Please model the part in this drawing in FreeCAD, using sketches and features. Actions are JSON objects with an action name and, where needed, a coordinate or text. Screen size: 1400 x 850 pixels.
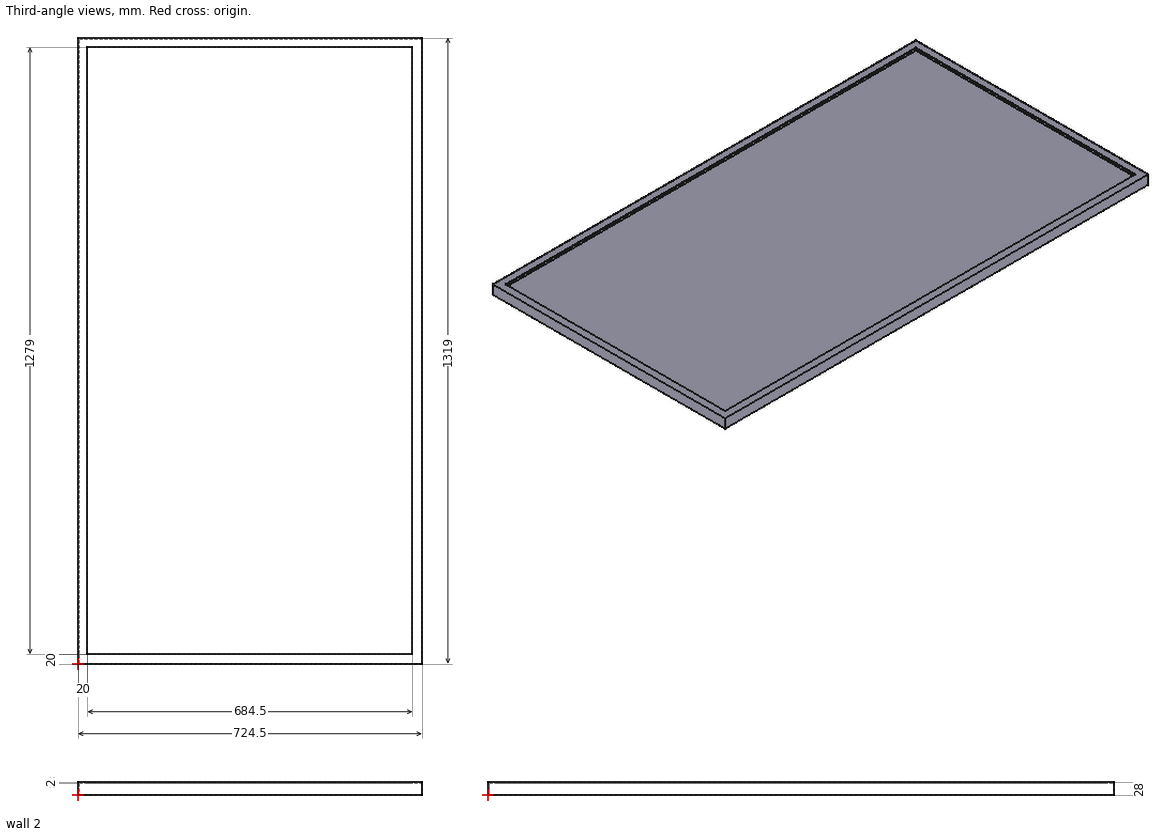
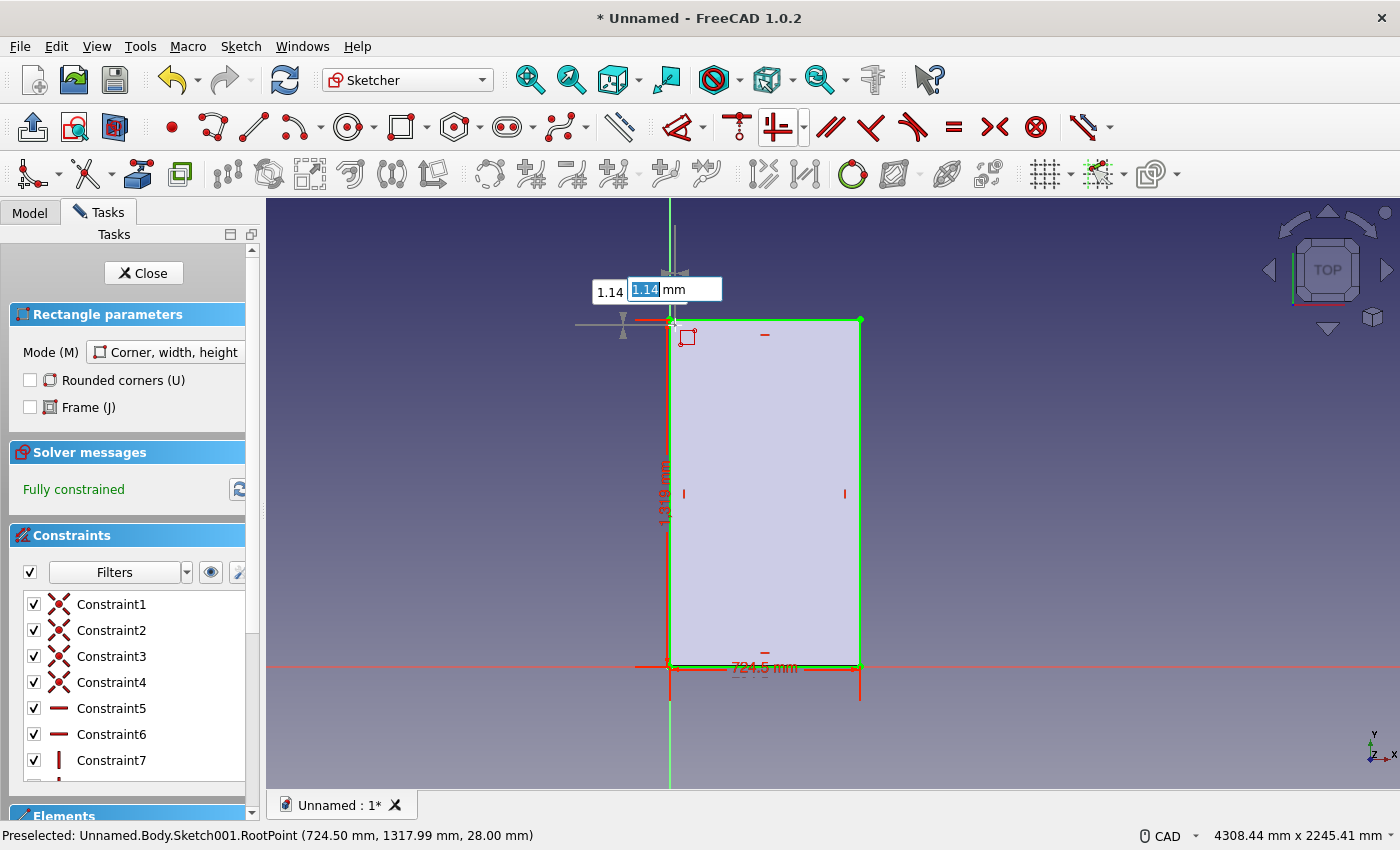
{"action": "scroll", "coordinate": [855, 662], "scroll_direction": "up", "scroll_amount": 6}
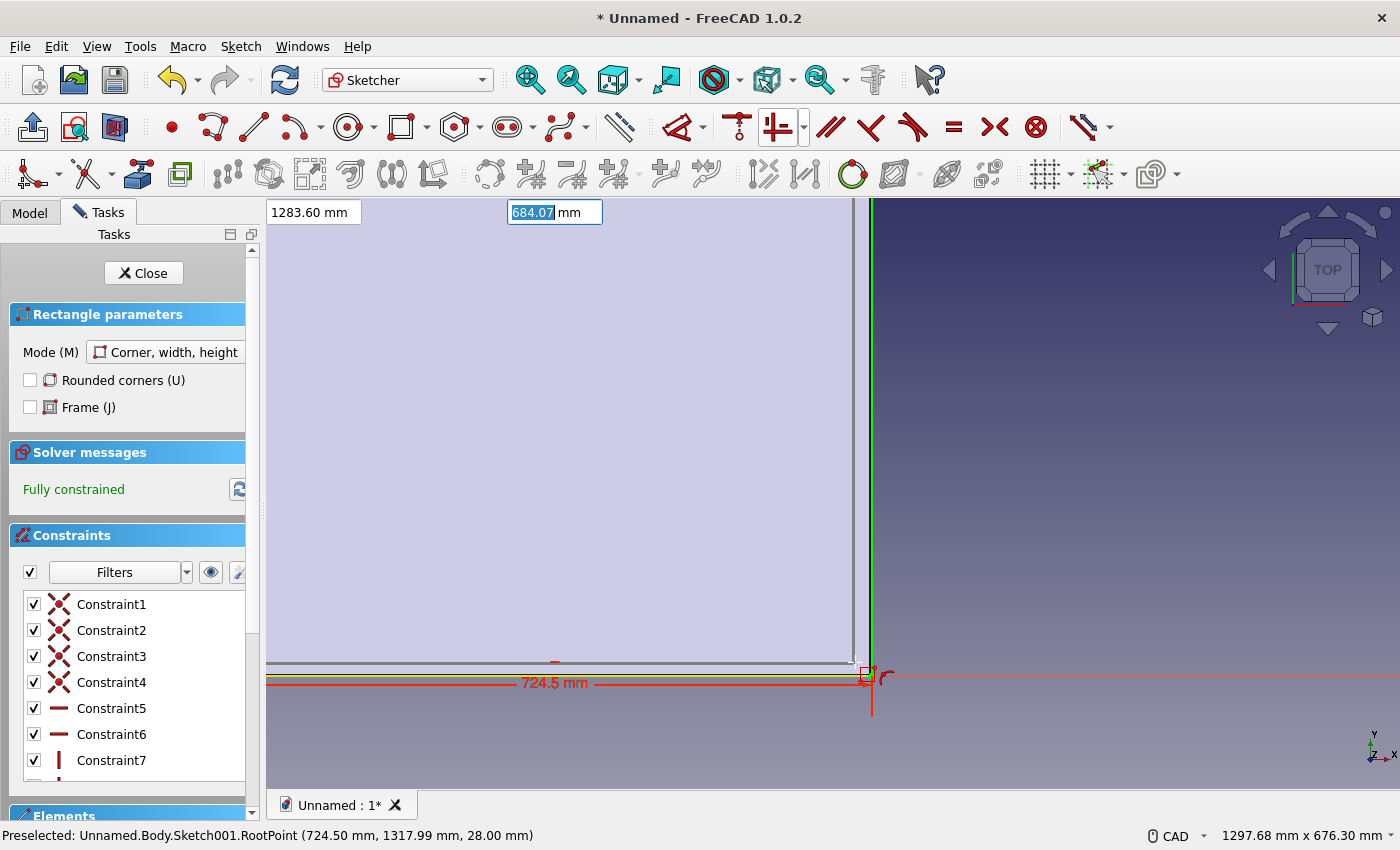
{"action": "left_click", "coordinate": [854, 659]}
{"action": "key", "text": "Escape"}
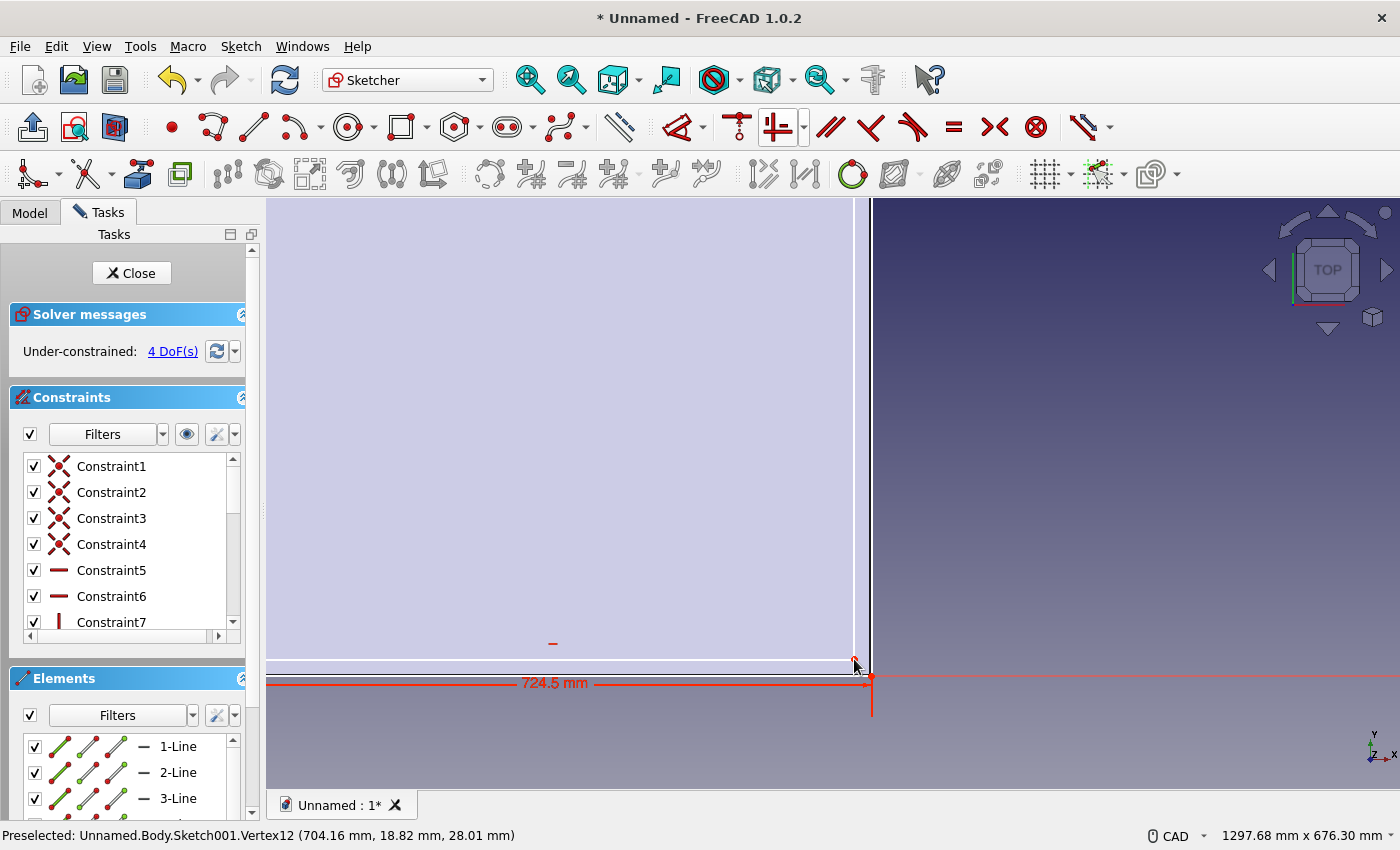
{"action": "left_click", "coordinate": [676, 128]}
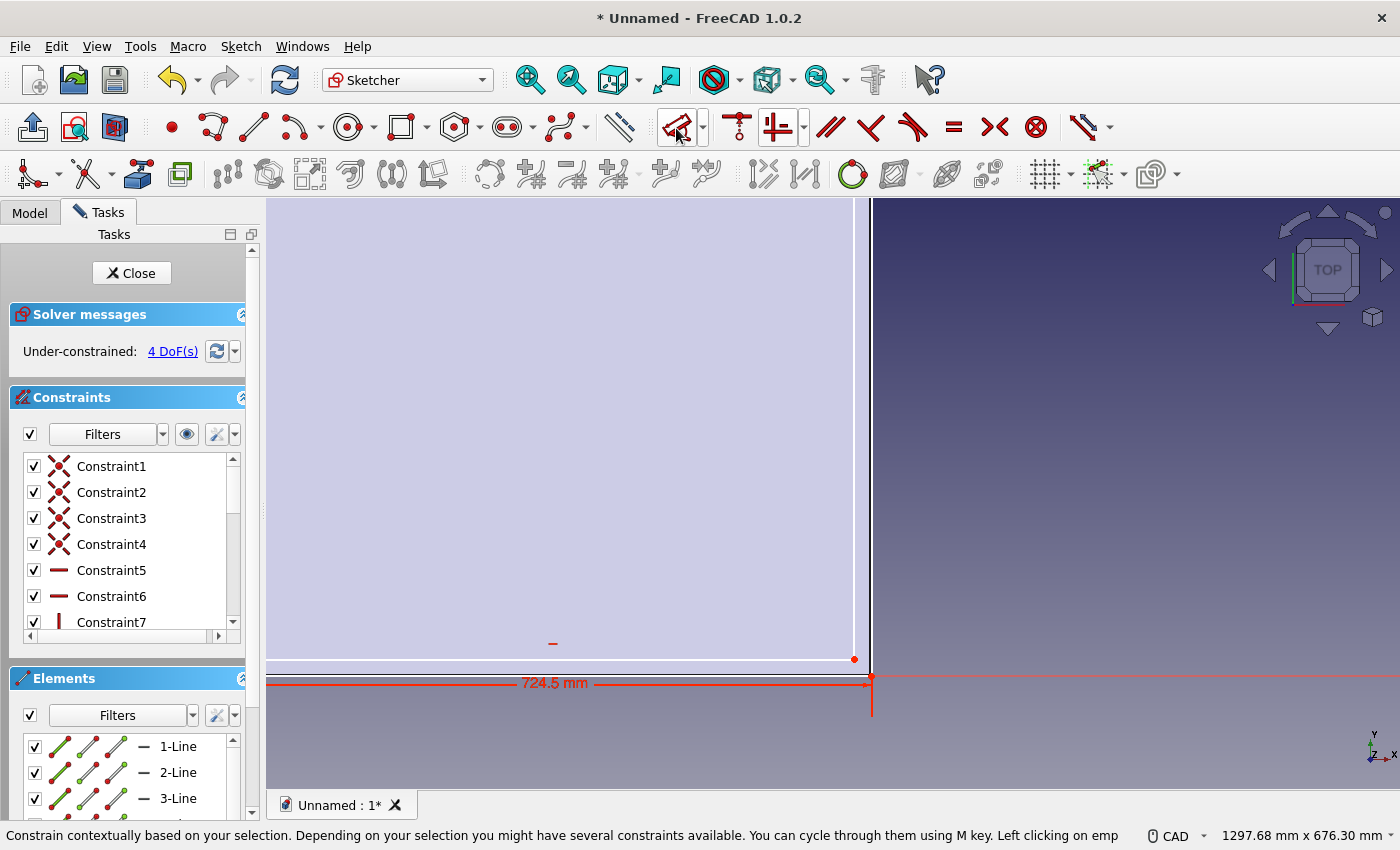
{"action": "scroll", "coordinate": [855, 663], "scroll_direction": "down", "scroll_amount": 6}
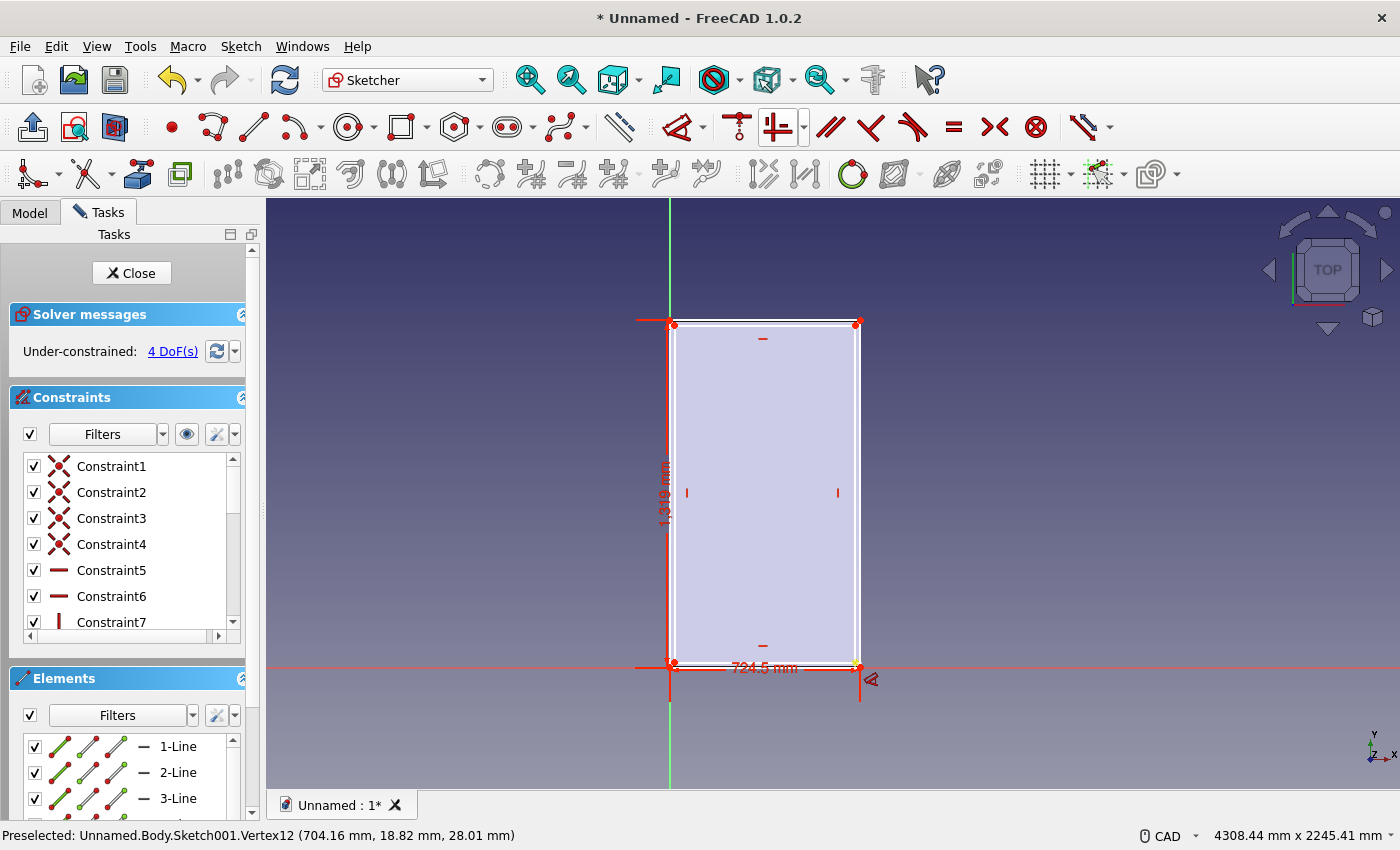
{"action": "scroll", "coordinate": [675, 326], "scroll_direction": "up", "scroll_amount": 11}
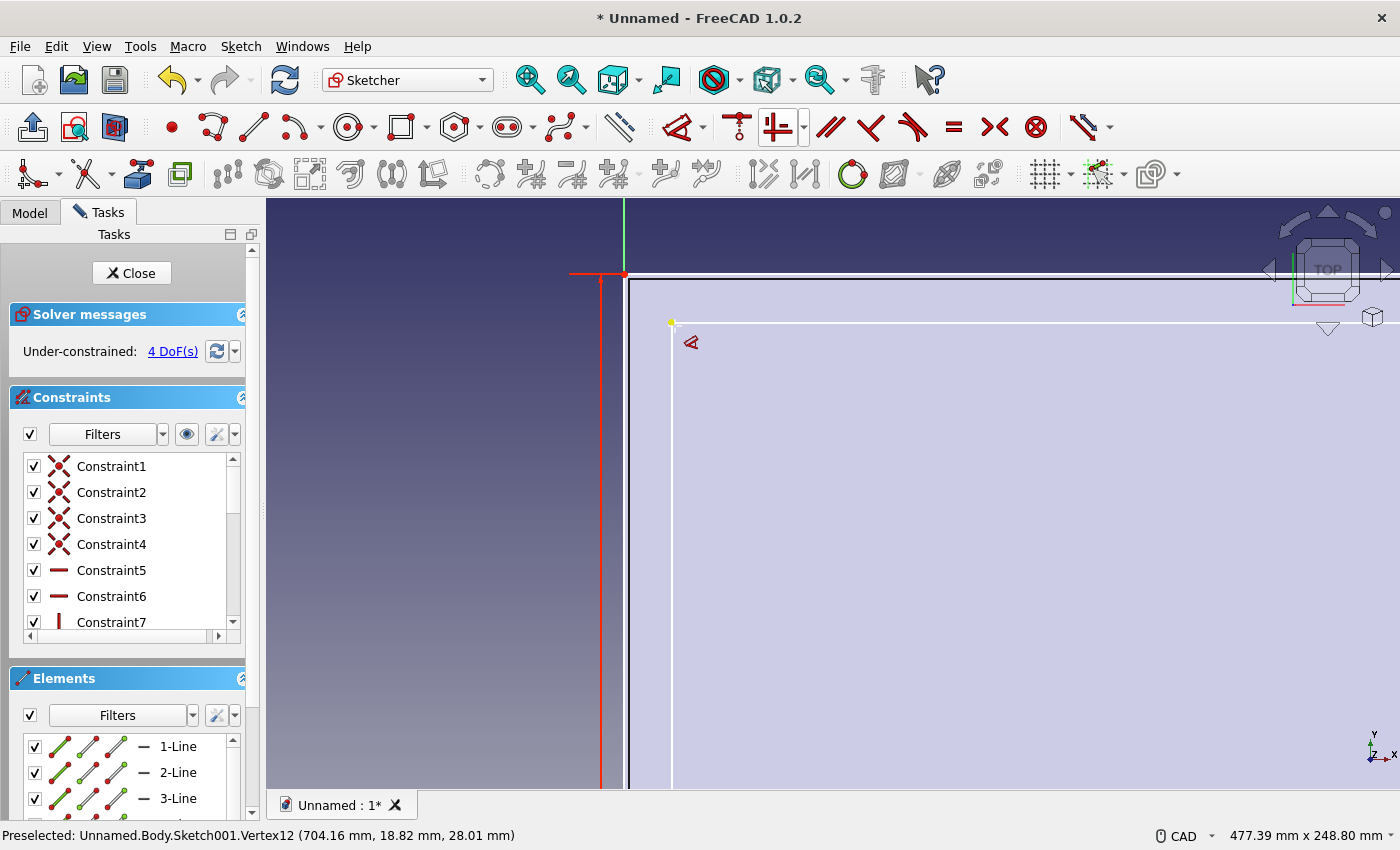
{"action": "left_click", "coordinate": [672, 323]}
{"action": "left_click", "coordinate": [648, 289]}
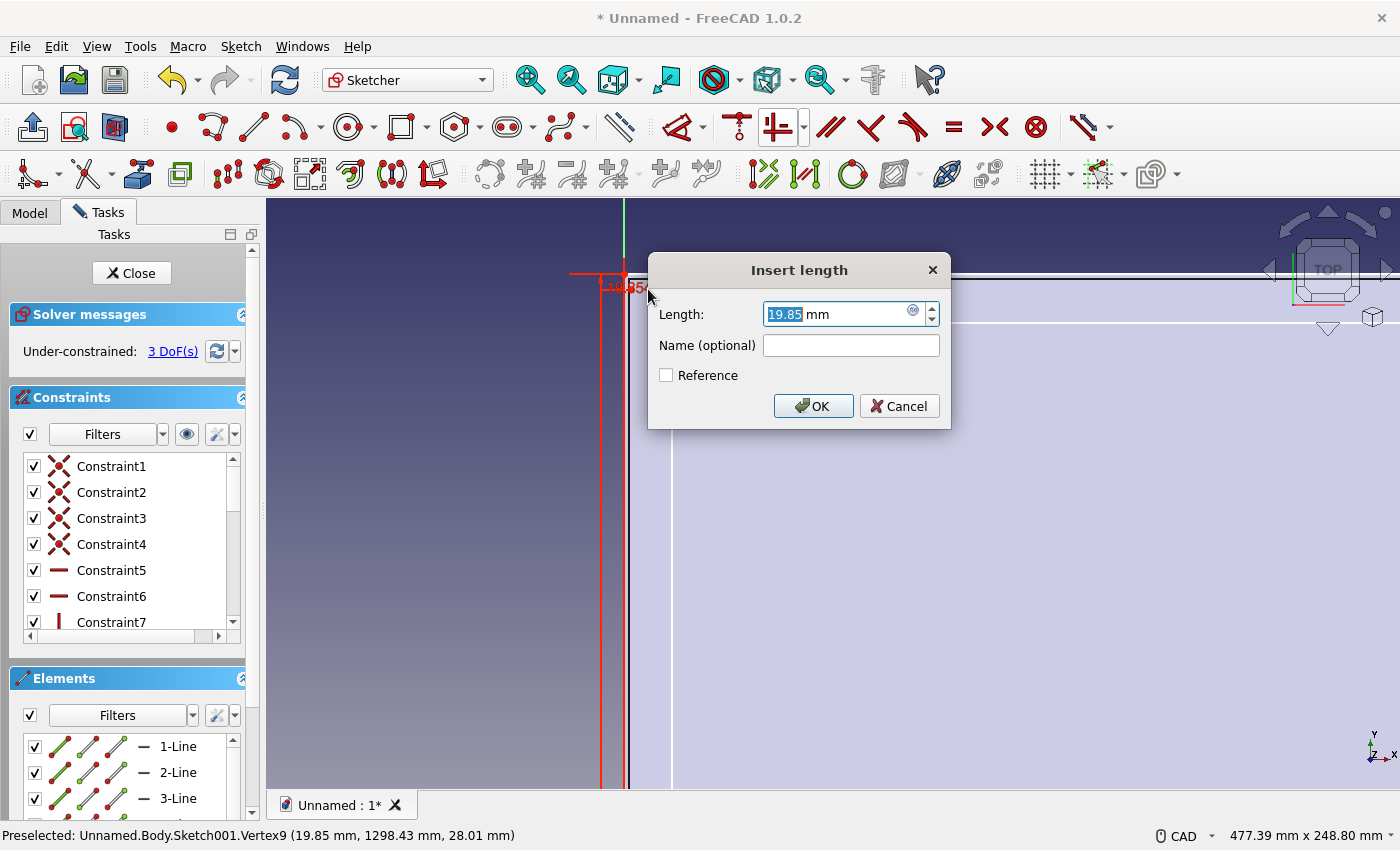
{"action": "type", "text": "20"}
{"action": "key", "text": "Return"}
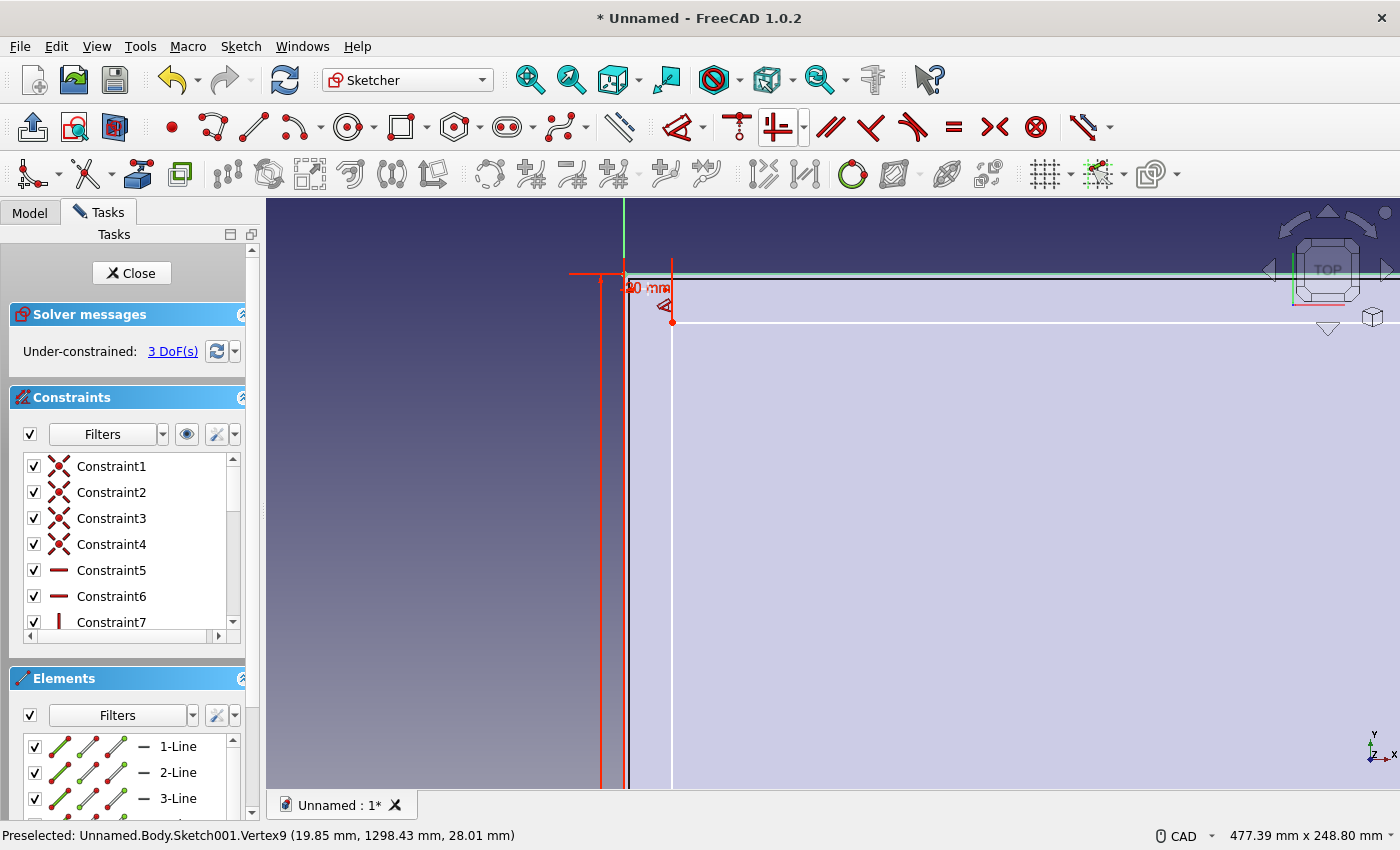
{"action": "scroll", "coordinate": [675, 326], "scroll_direction": "down", "scroll_amount": 11}